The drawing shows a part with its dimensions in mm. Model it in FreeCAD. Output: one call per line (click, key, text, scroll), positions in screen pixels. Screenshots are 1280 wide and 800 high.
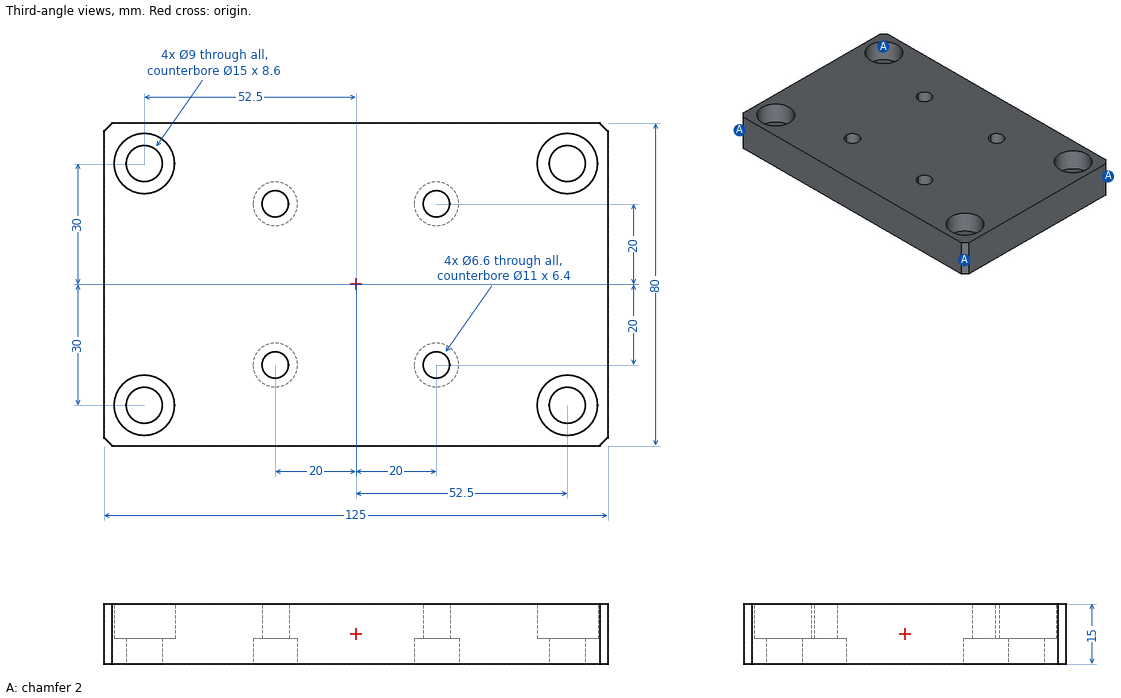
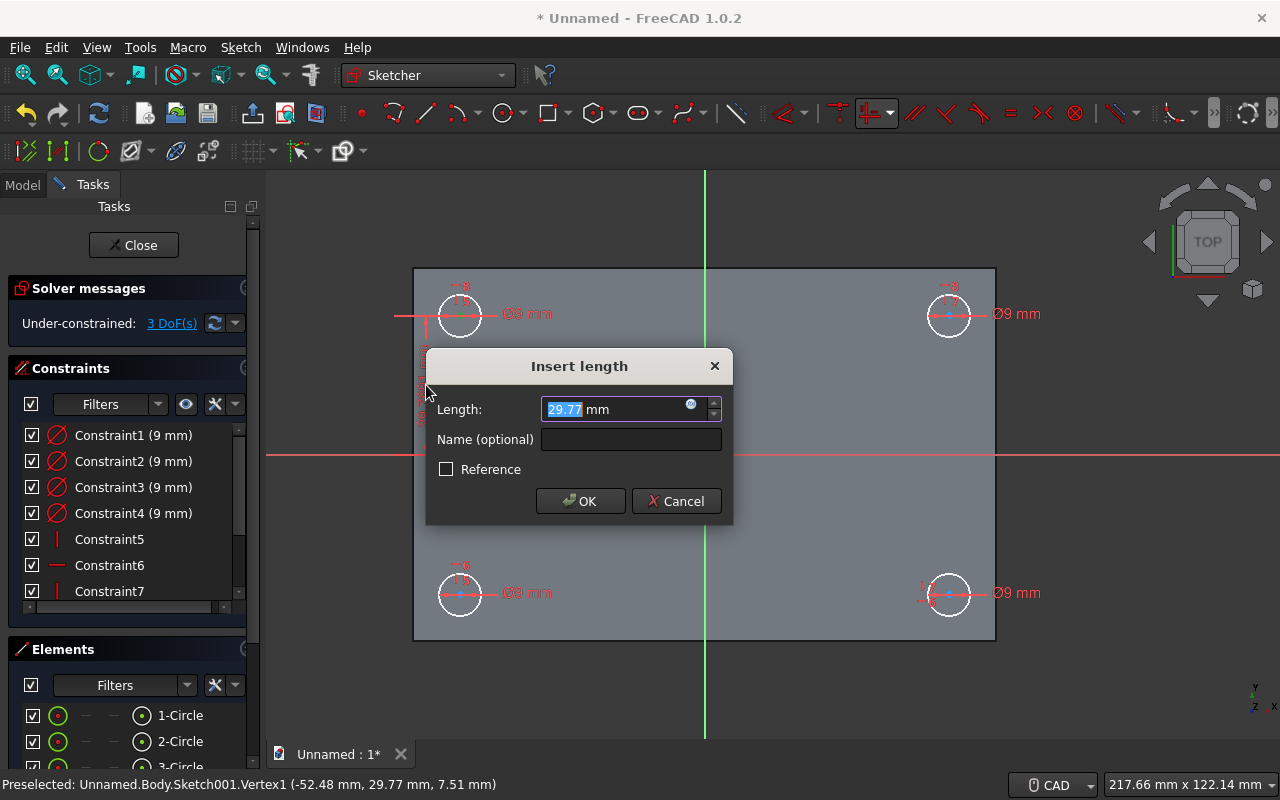
text(30)
key(Return)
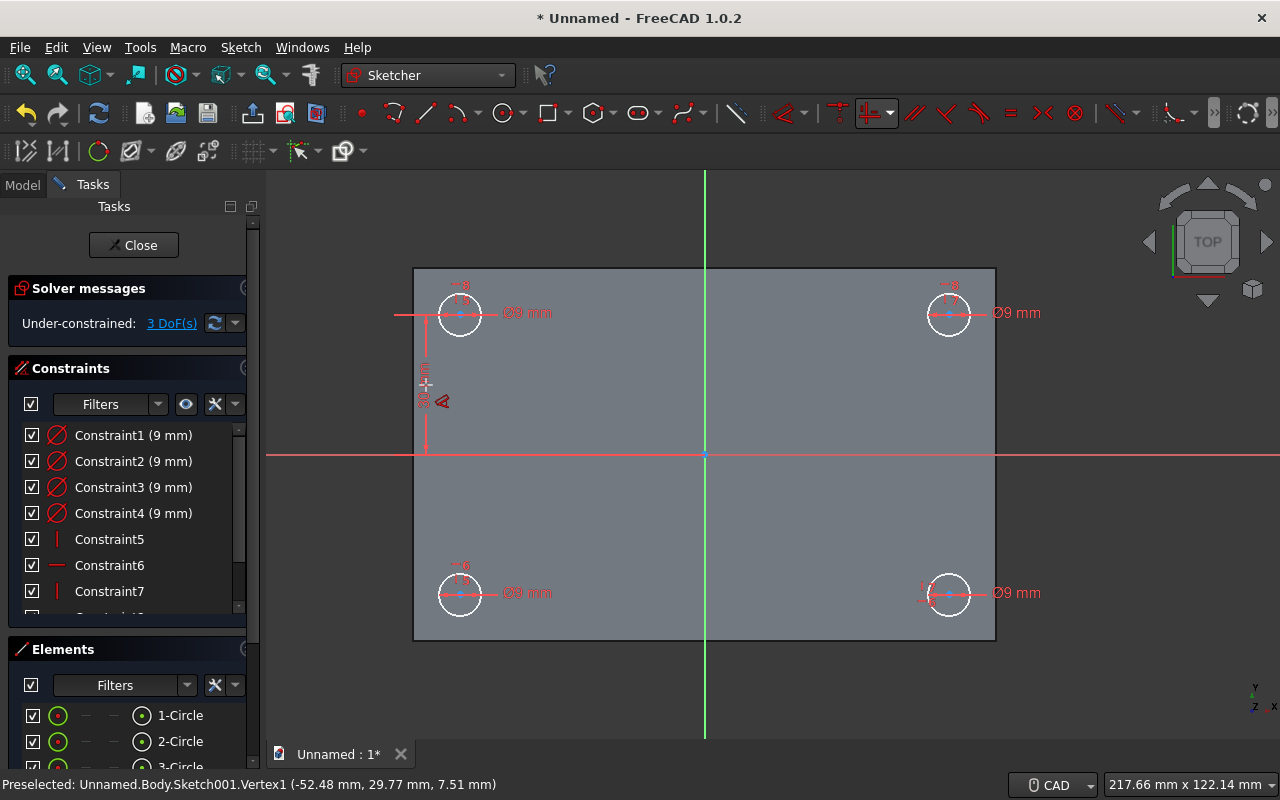
click(460, 595)
click(426, 525)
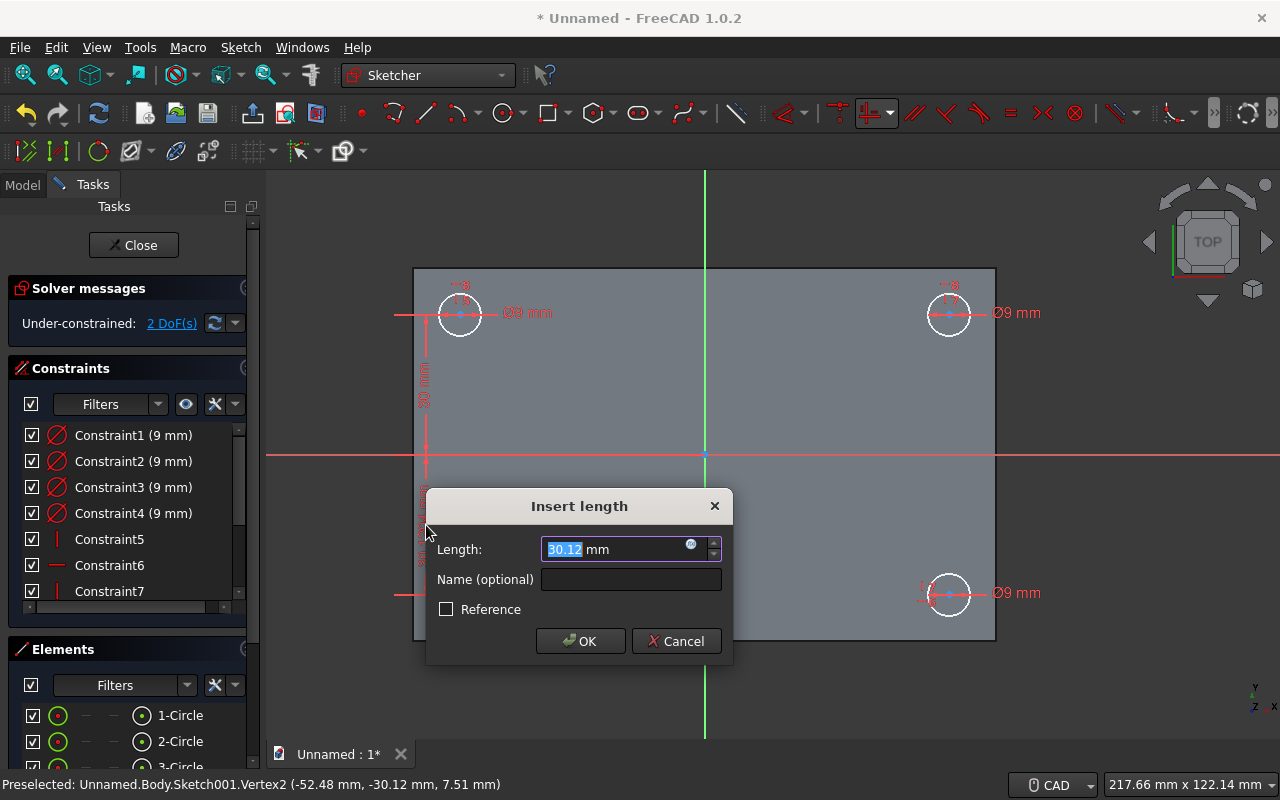
text(30)
key(Return)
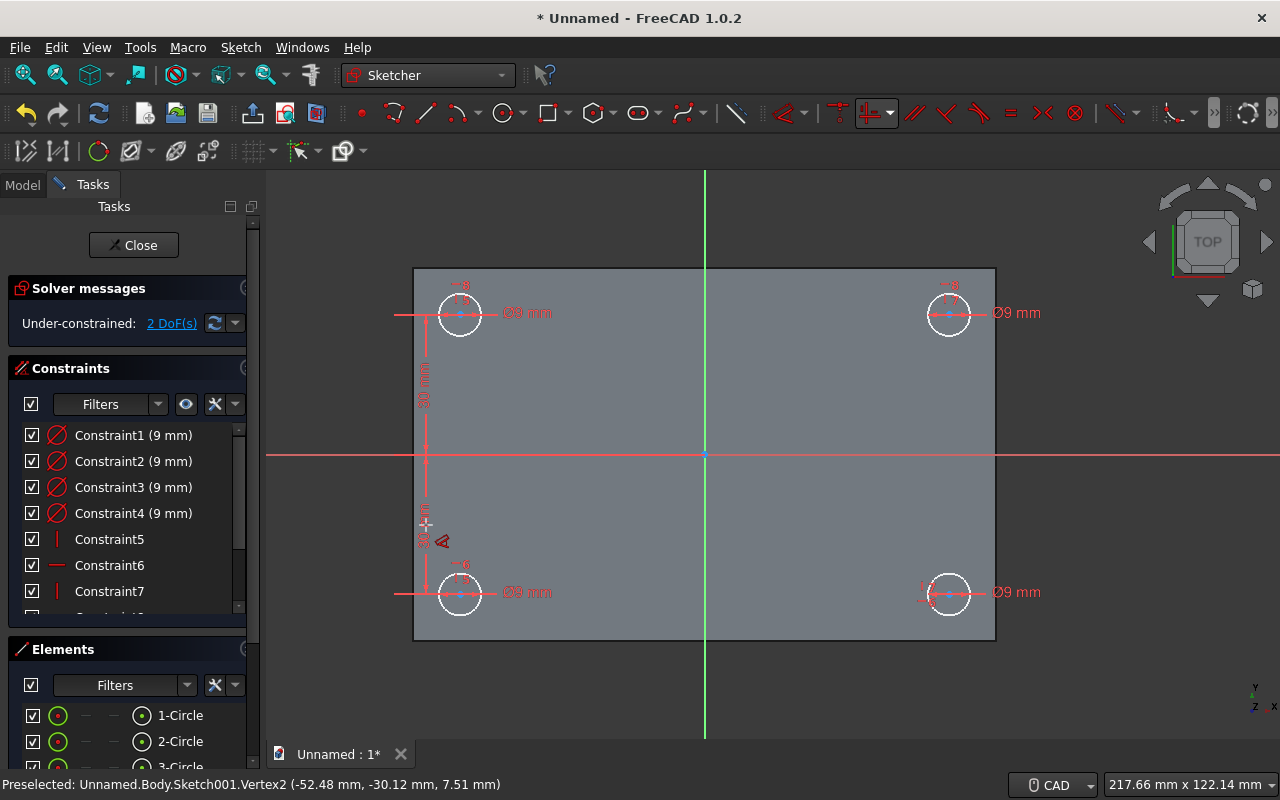
click(460, 315)
click(582, 281)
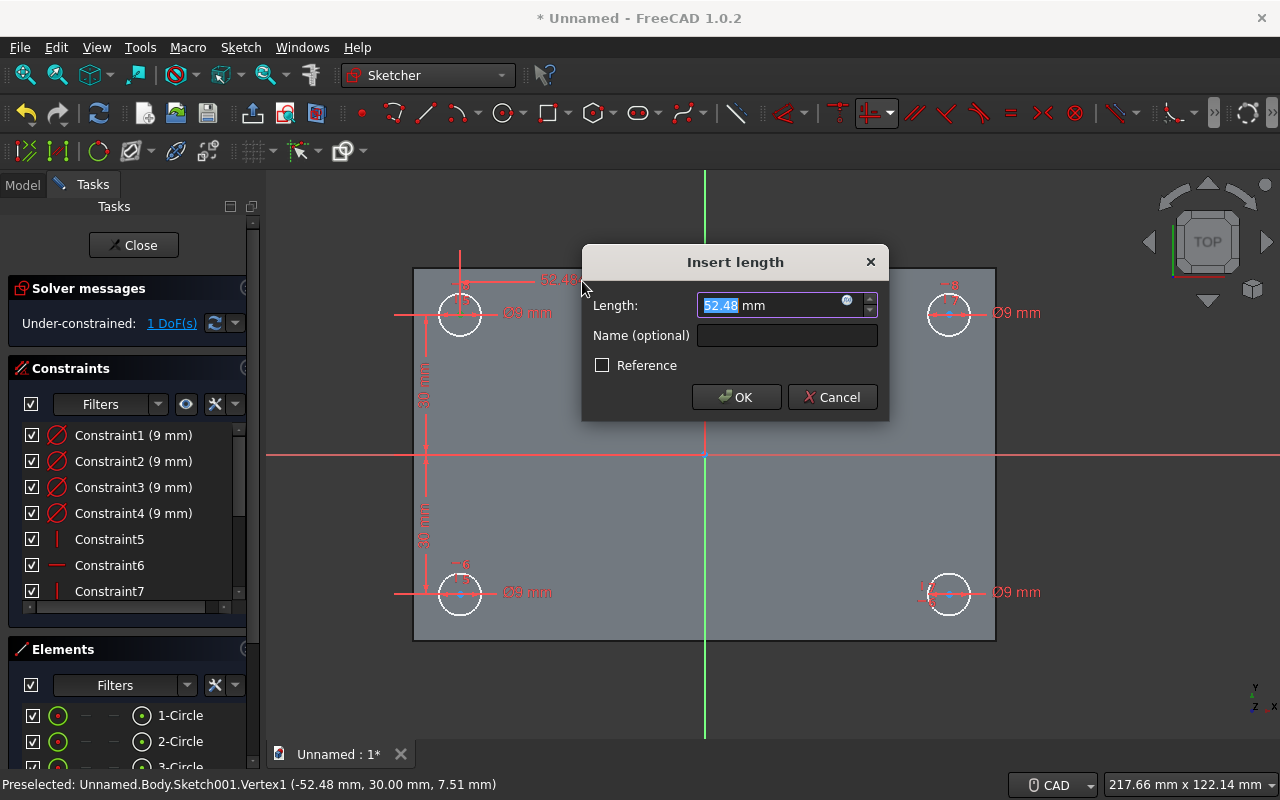
text(52.5)
key(Return)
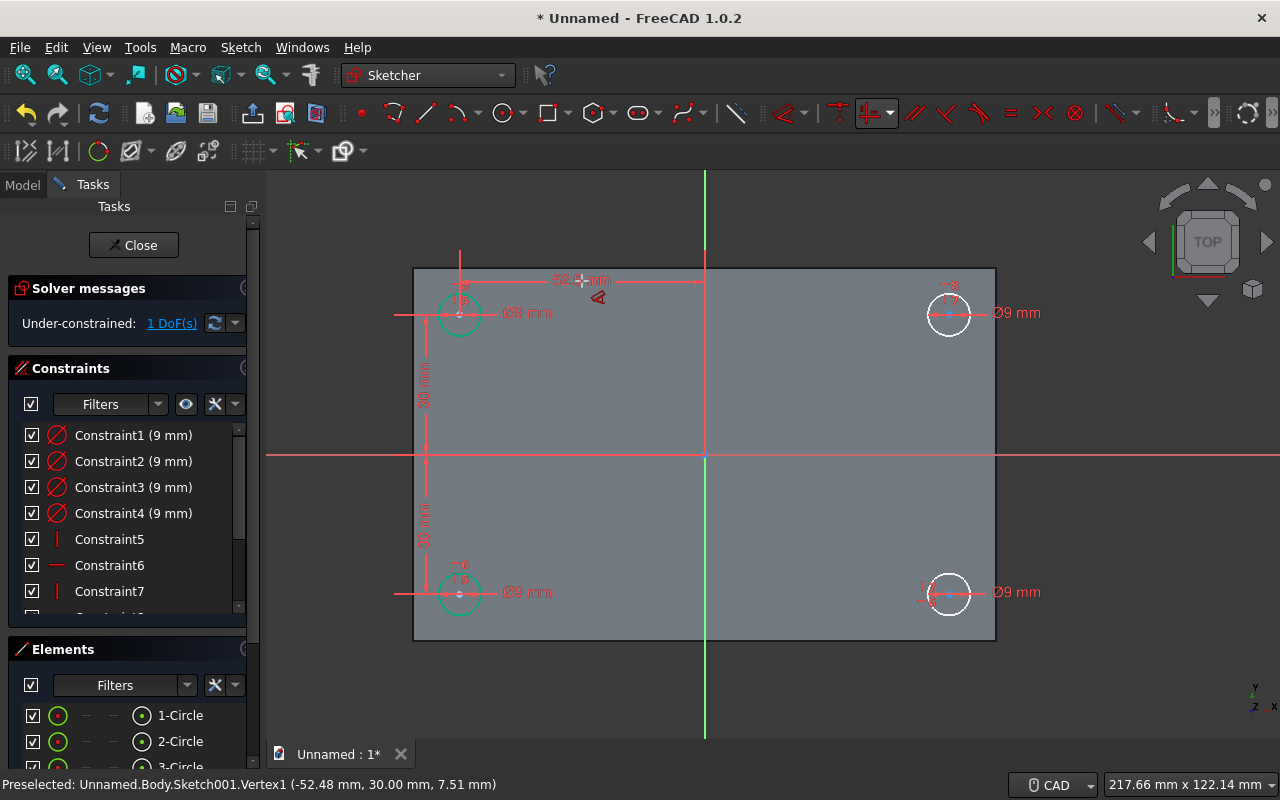
click(949, 594)
click(827, 628)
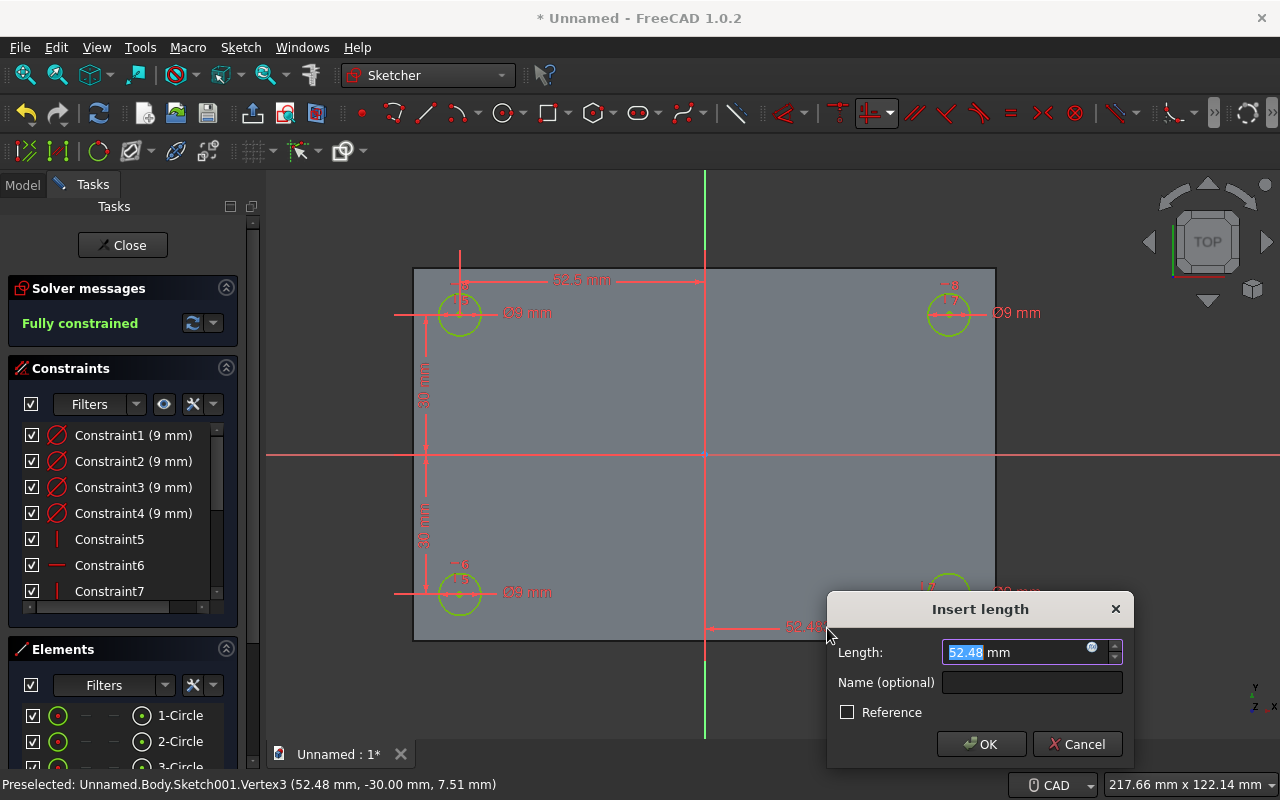
text(52.5)
key(Return)
key(Escape)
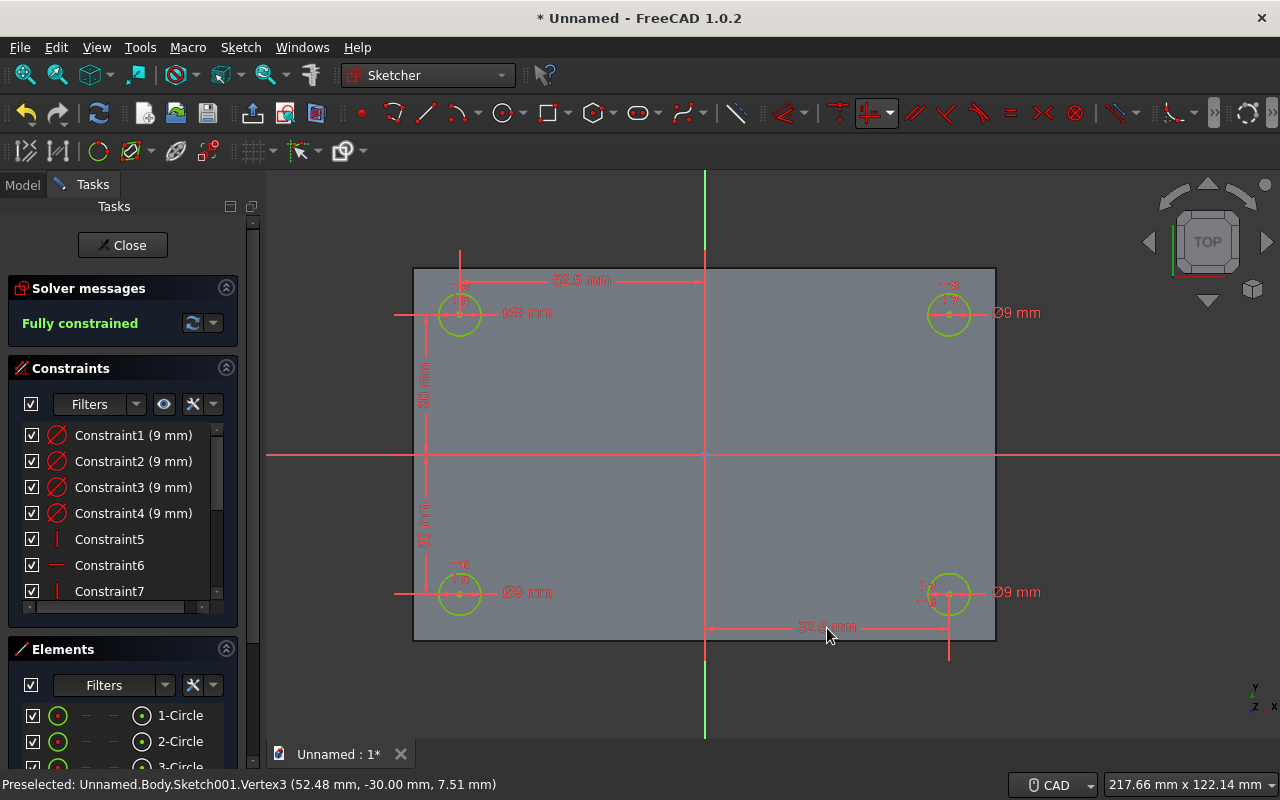
click(123, 245)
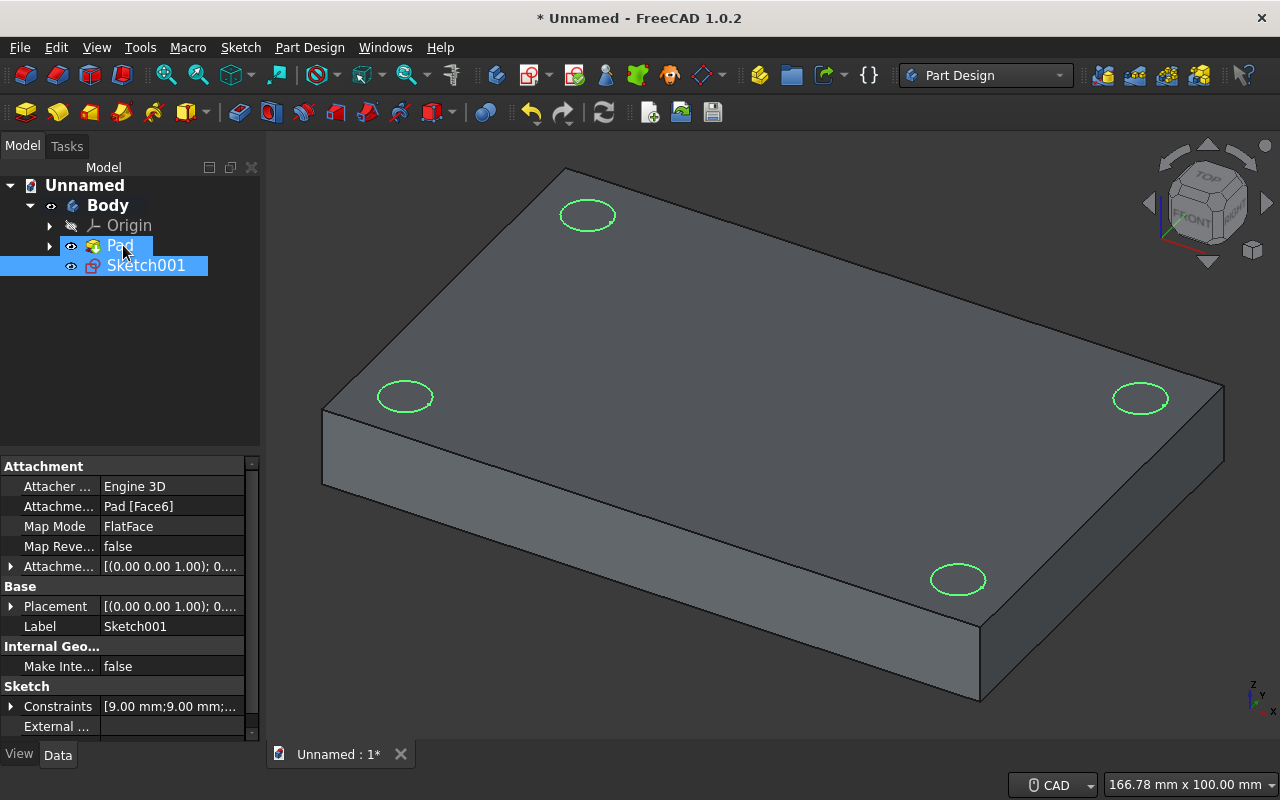
click(272, 112)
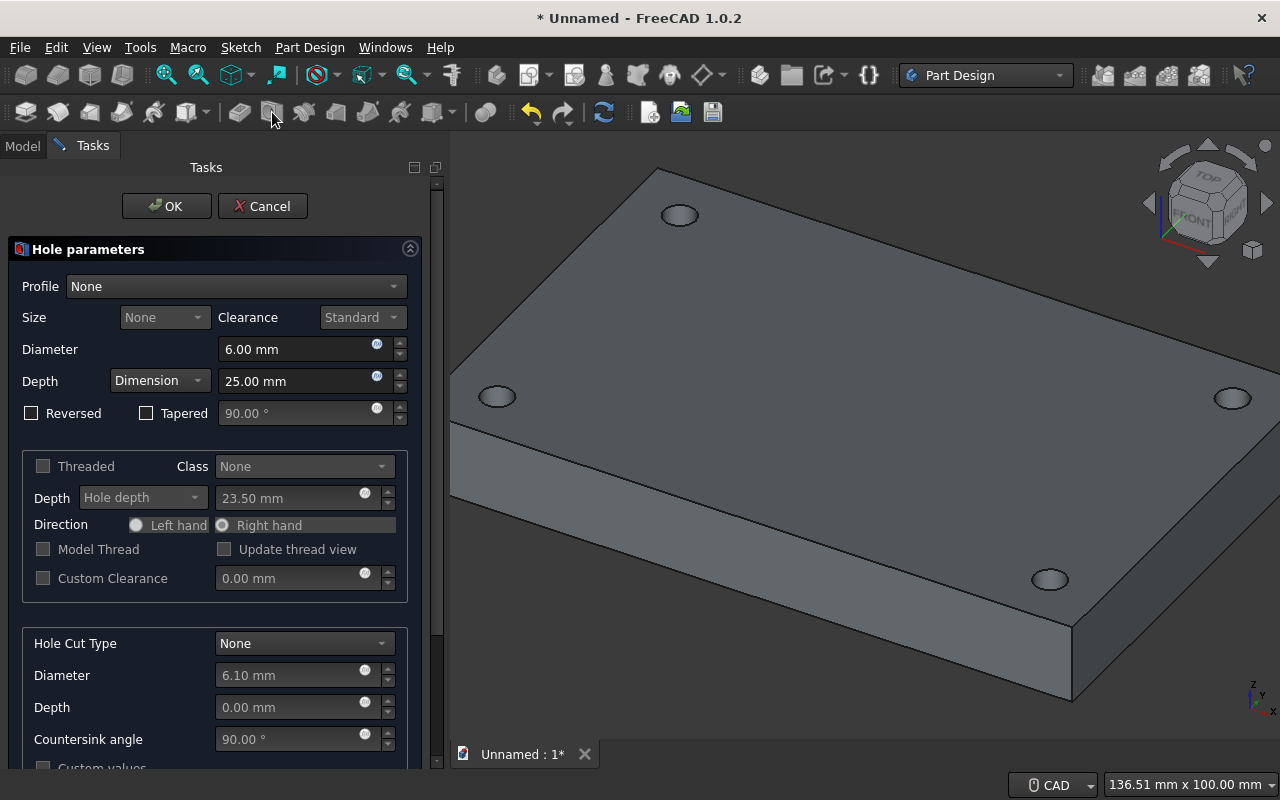
triple_click(305, 349)